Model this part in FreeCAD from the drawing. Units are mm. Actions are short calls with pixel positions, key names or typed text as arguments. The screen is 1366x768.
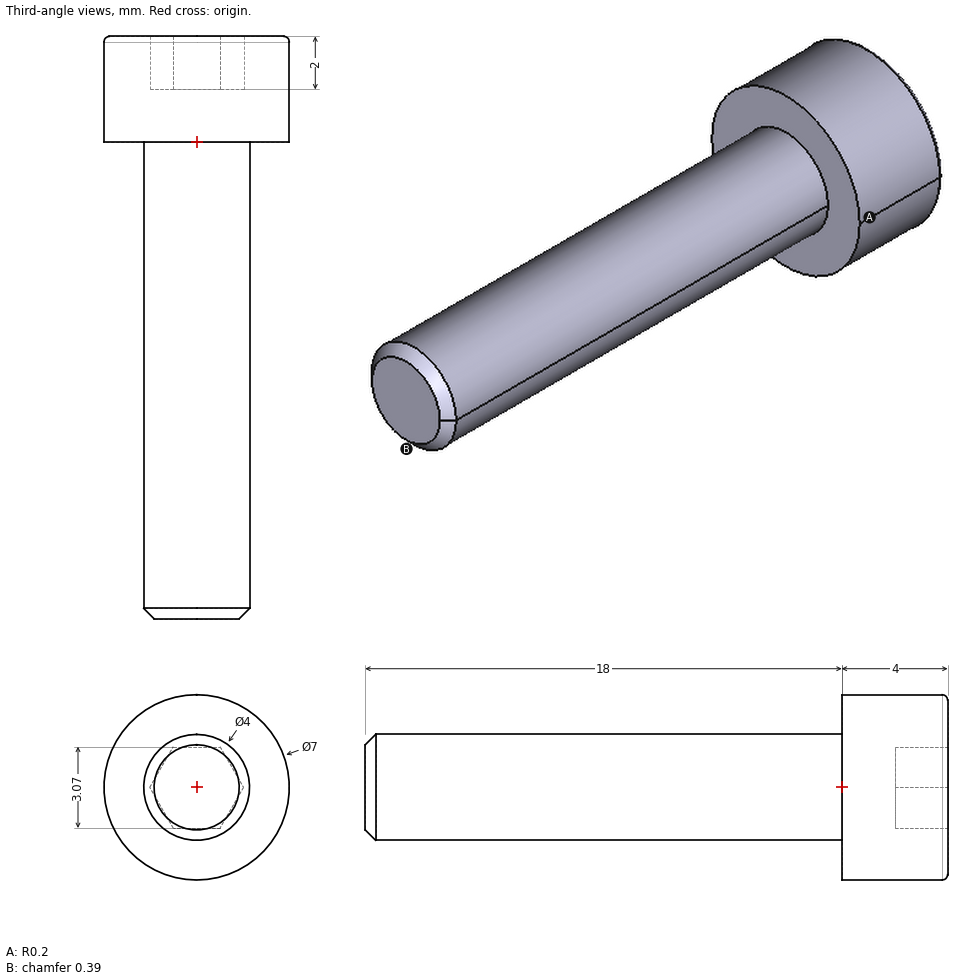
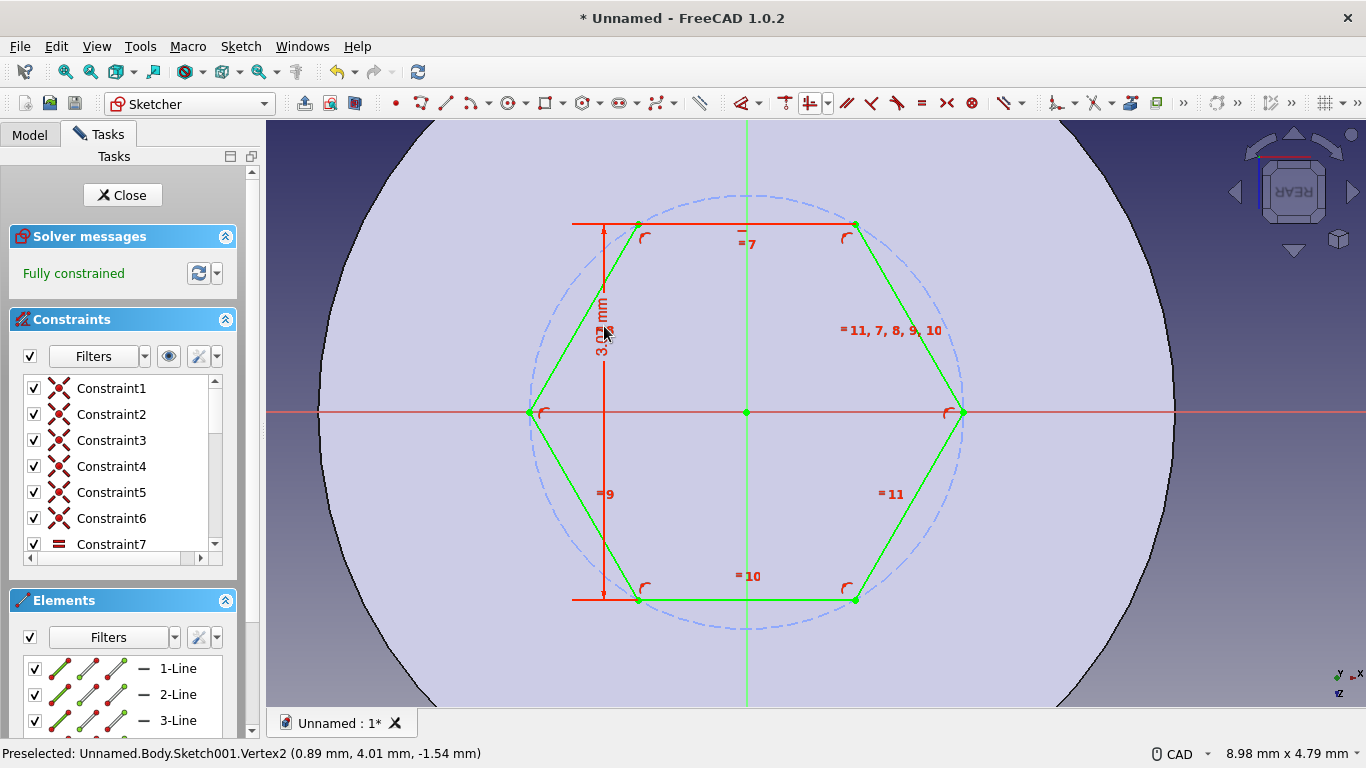
click(123, 195)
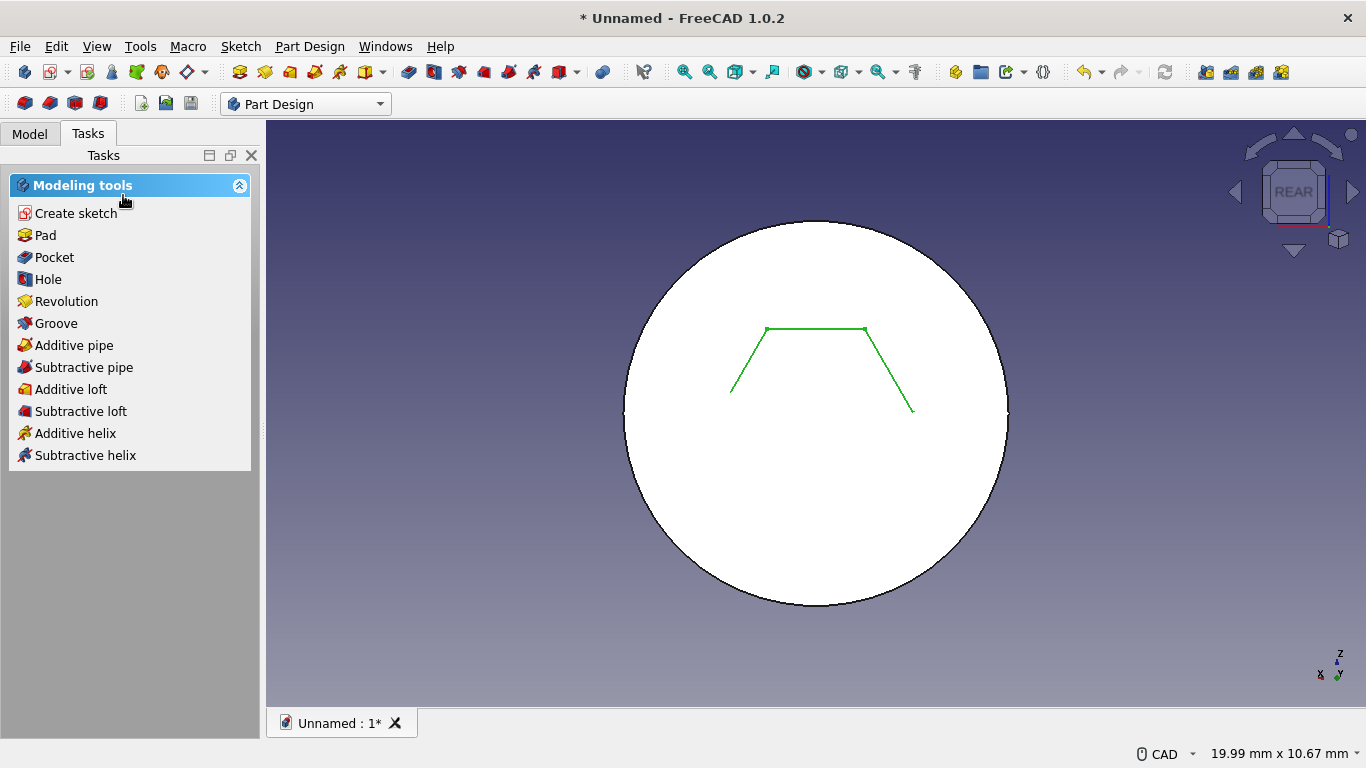
click(409, 72)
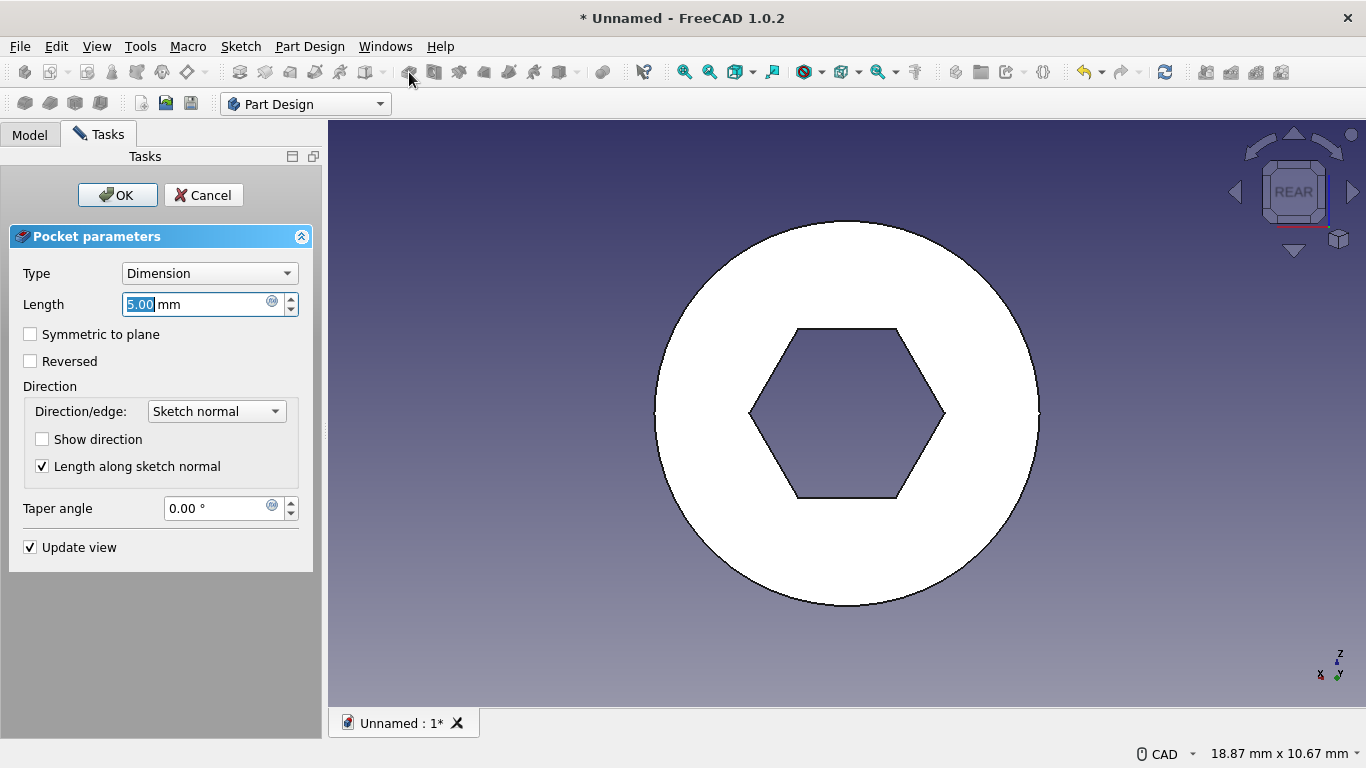
text(2)
key(Tab)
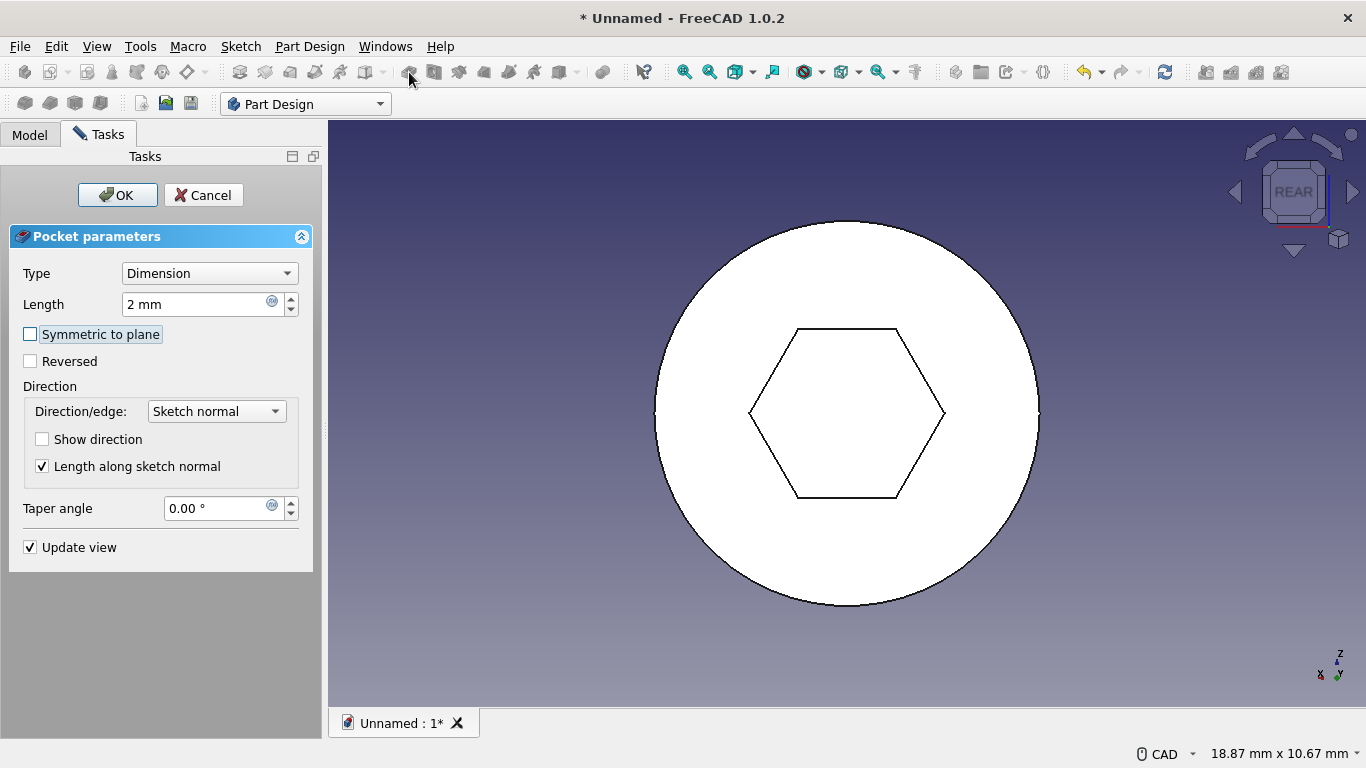
click(118, 195)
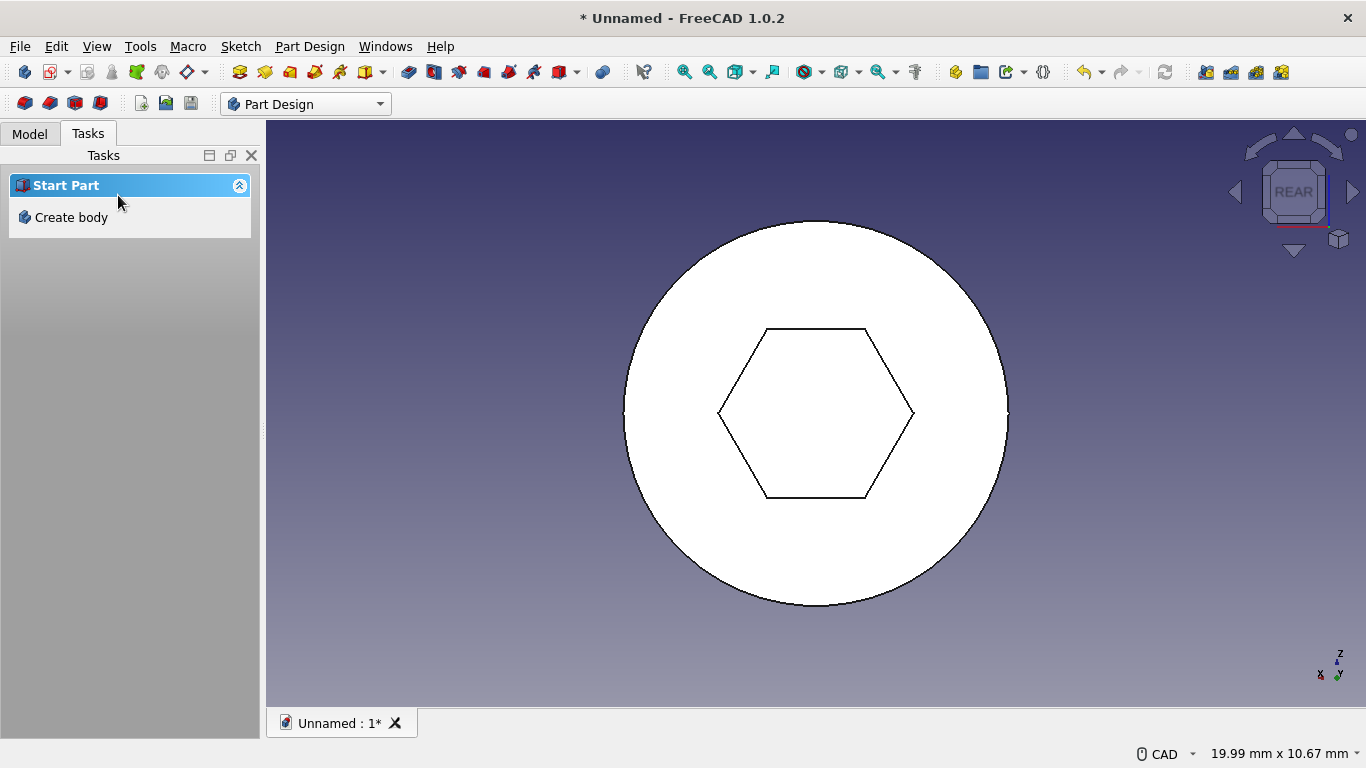
click(1009, 413)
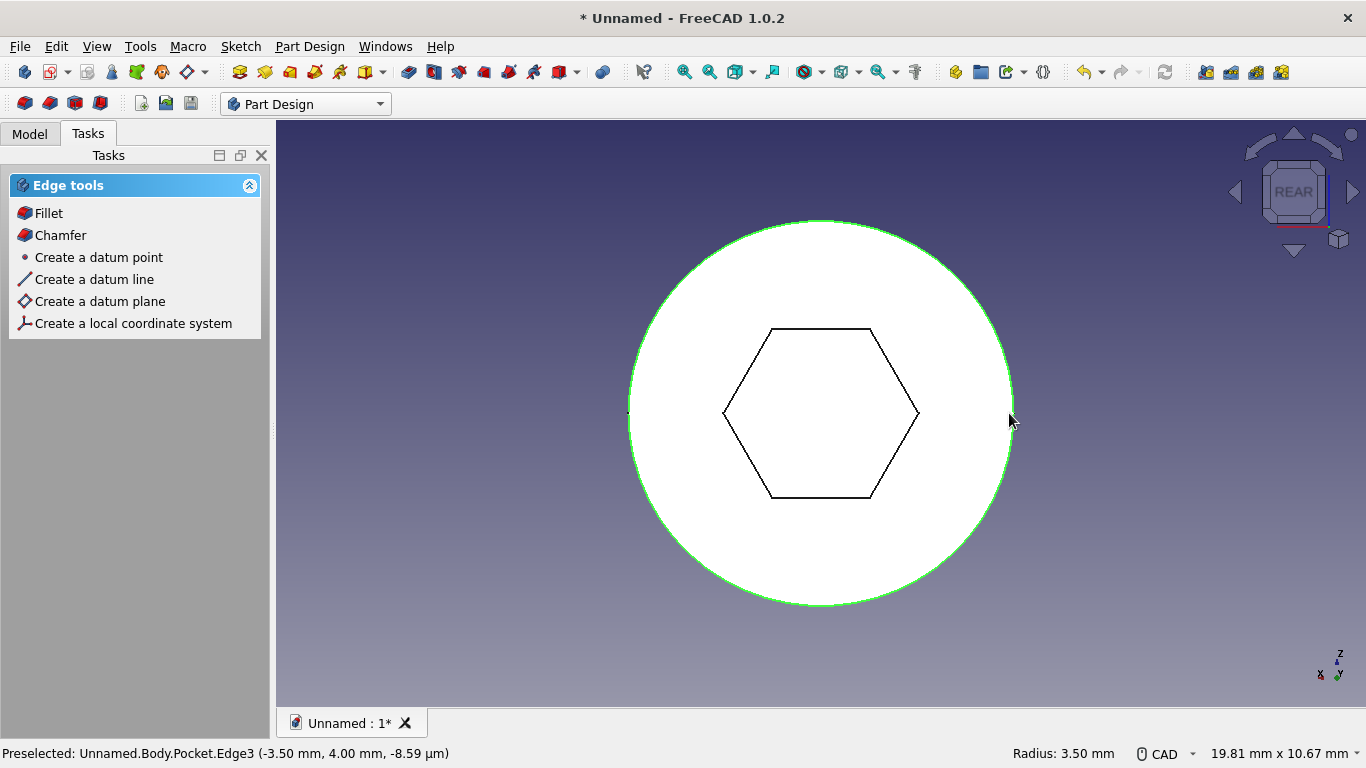
click(25, 104)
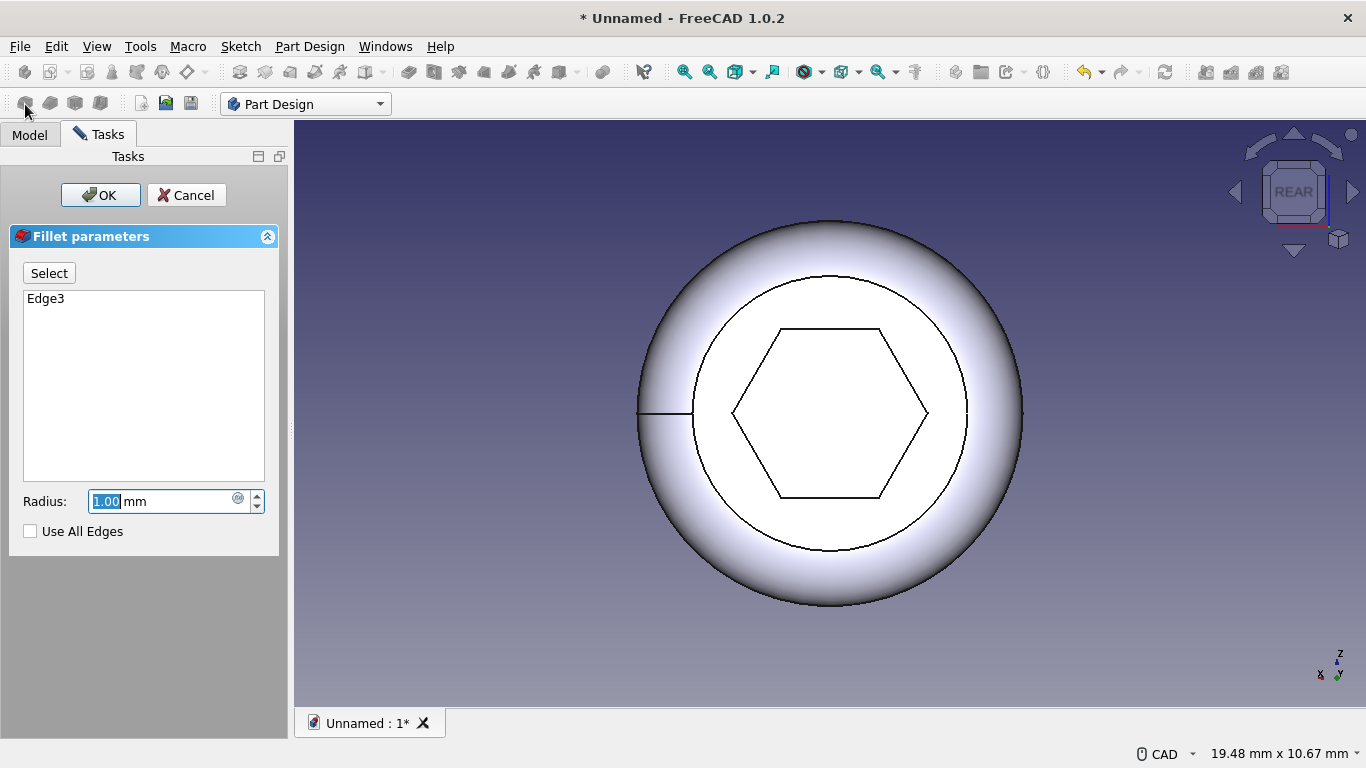
text(0.2)
key(Tab)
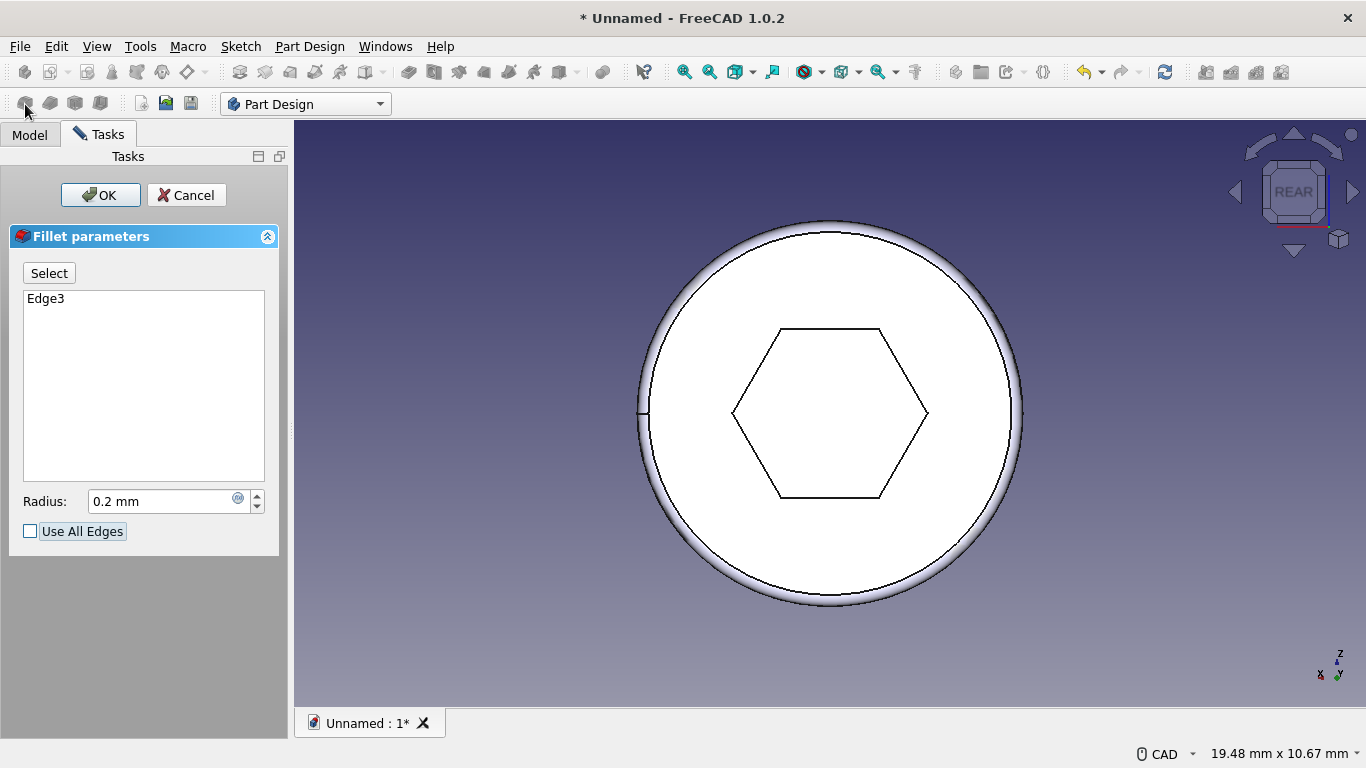
click(101, 195)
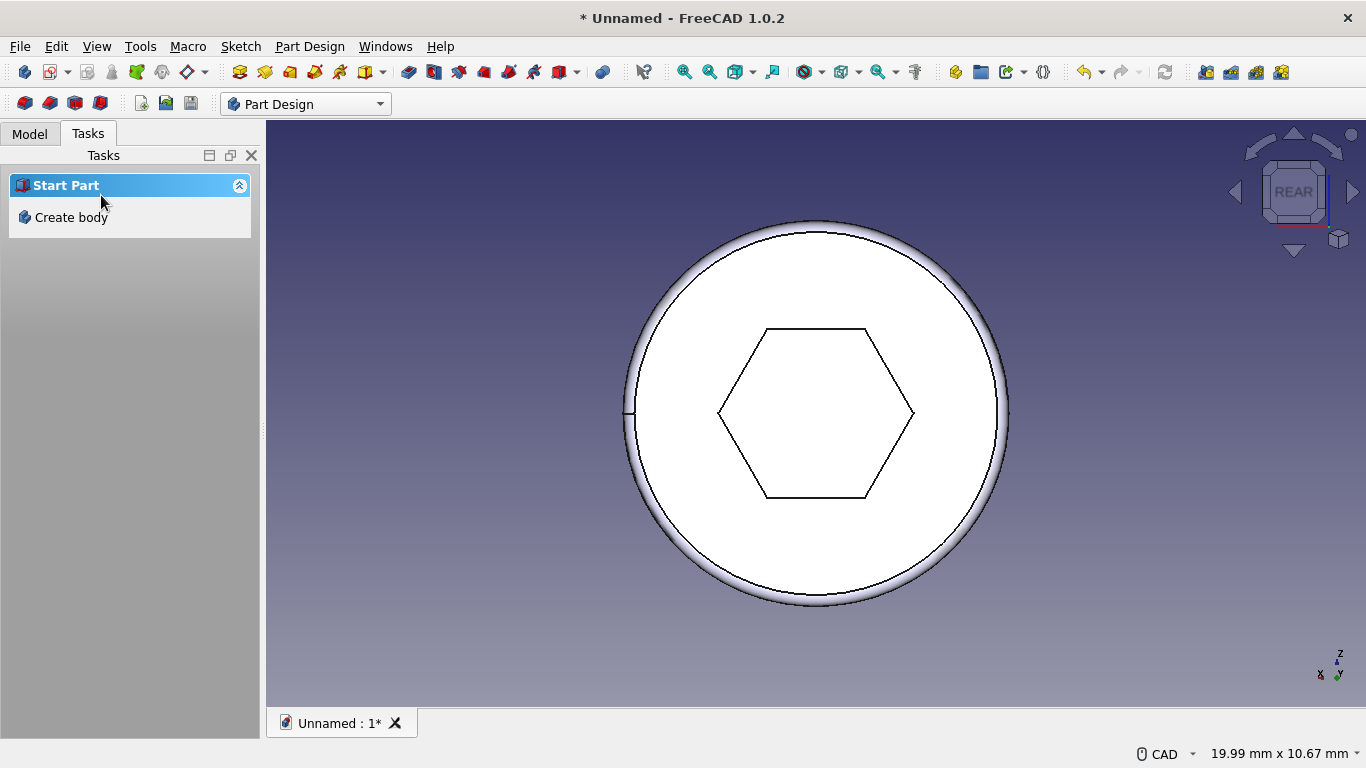
key(0)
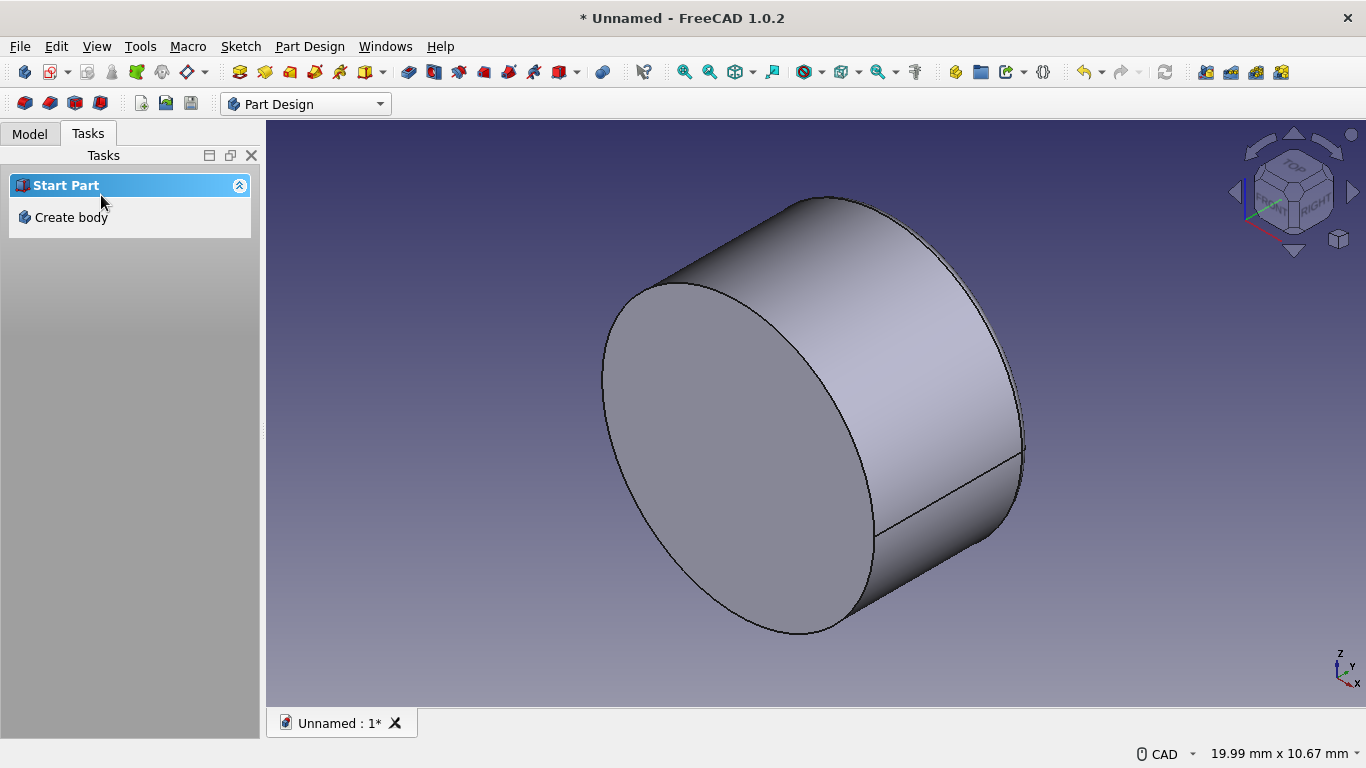
click(738, 457)